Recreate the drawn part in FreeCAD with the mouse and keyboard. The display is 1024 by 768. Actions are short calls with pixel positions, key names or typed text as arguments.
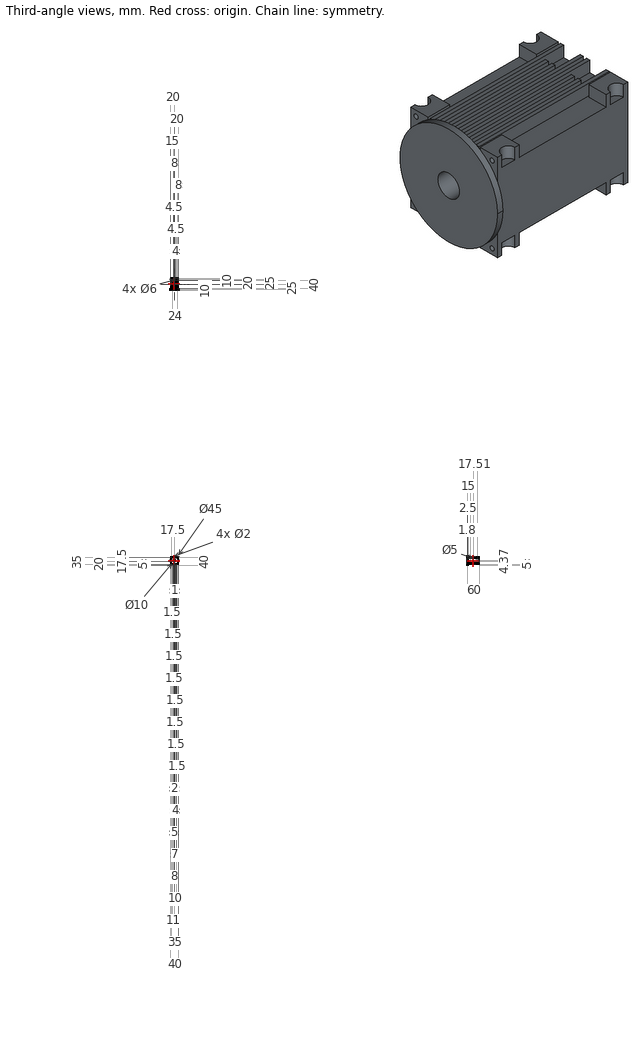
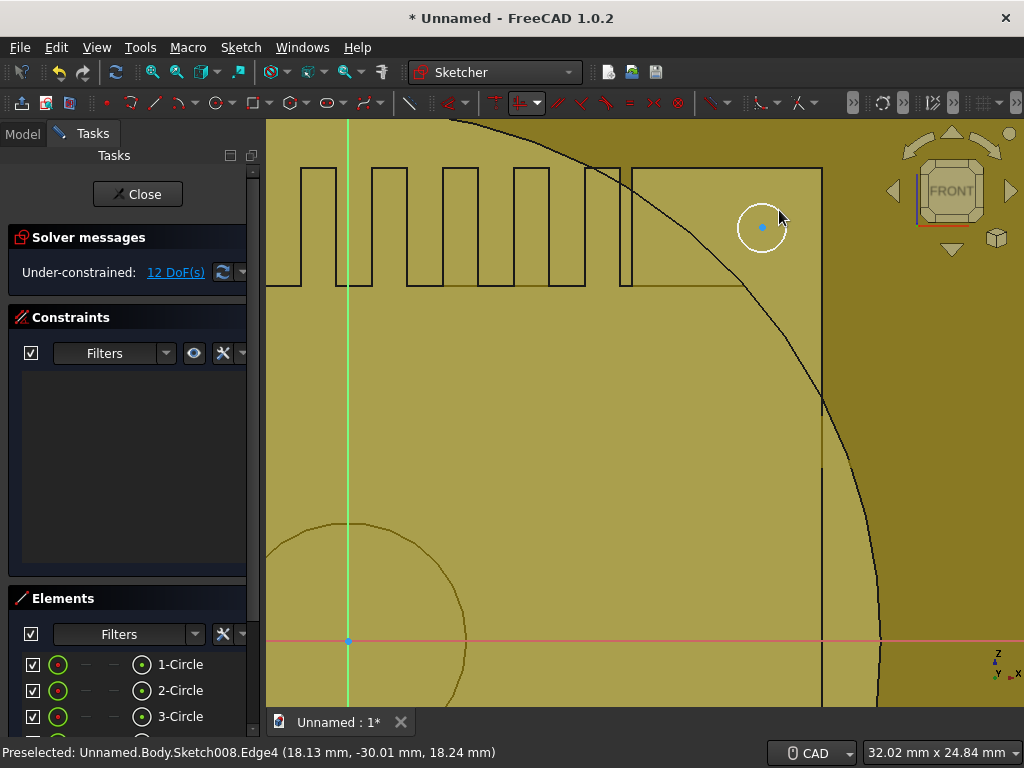
scroll(763, 227, down, 4)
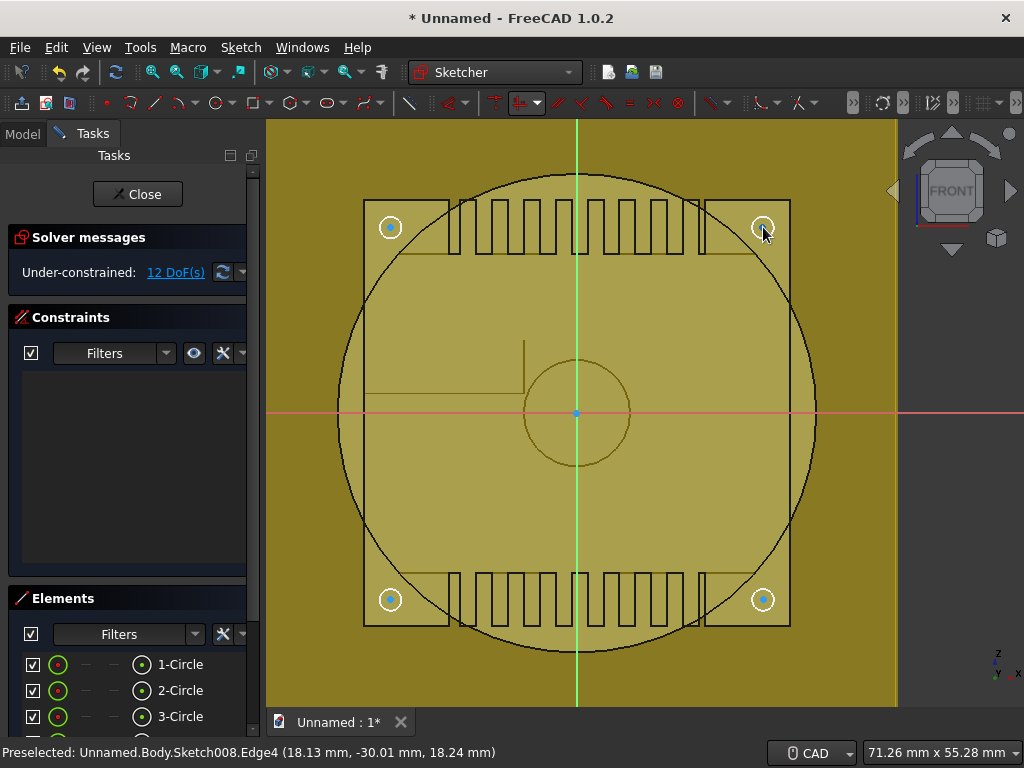
scroll(398, 220, up, 2)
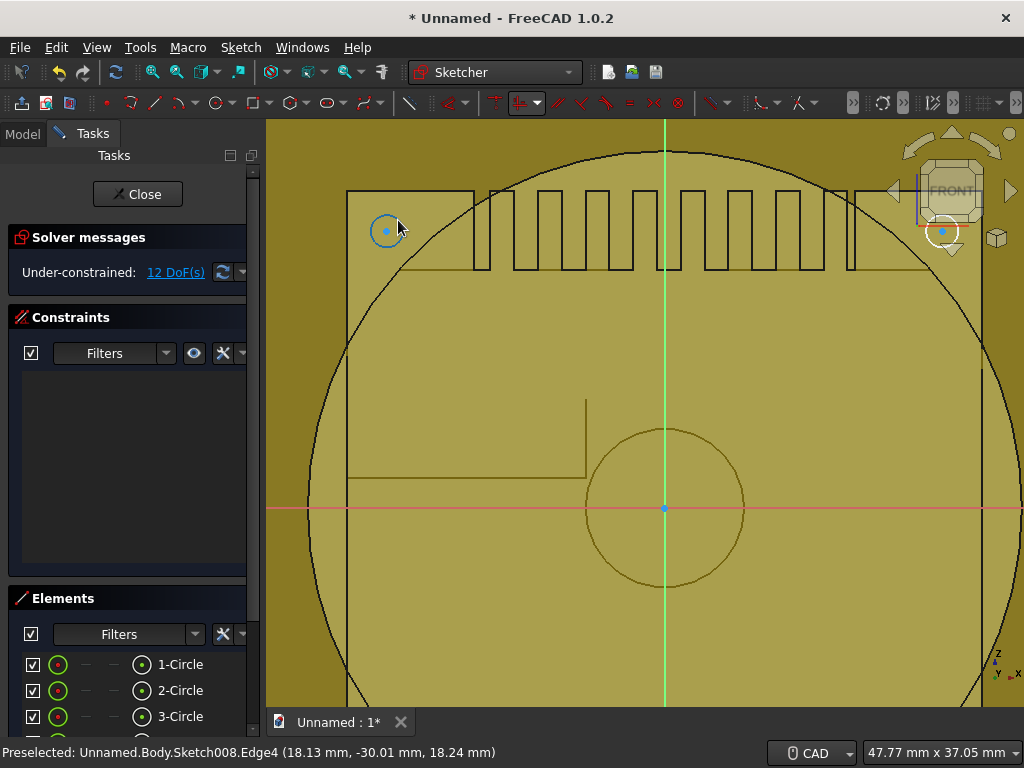
click(398, 220)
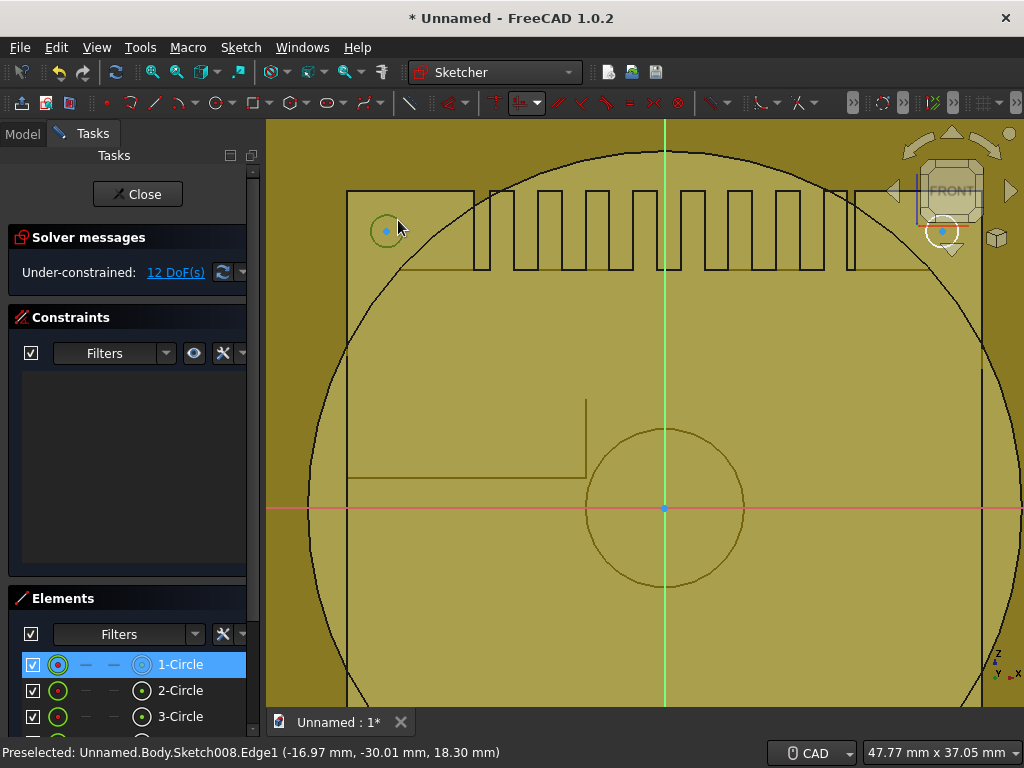
scroll(397, 220, down, 2)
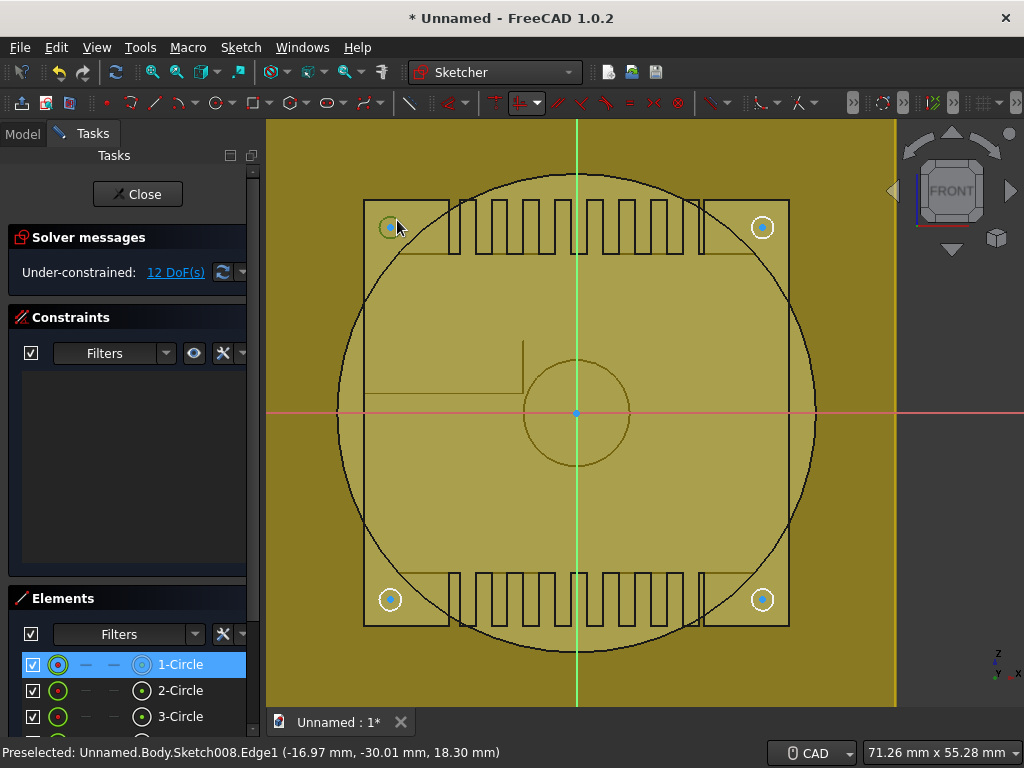
scroll(398, 592, up, 2)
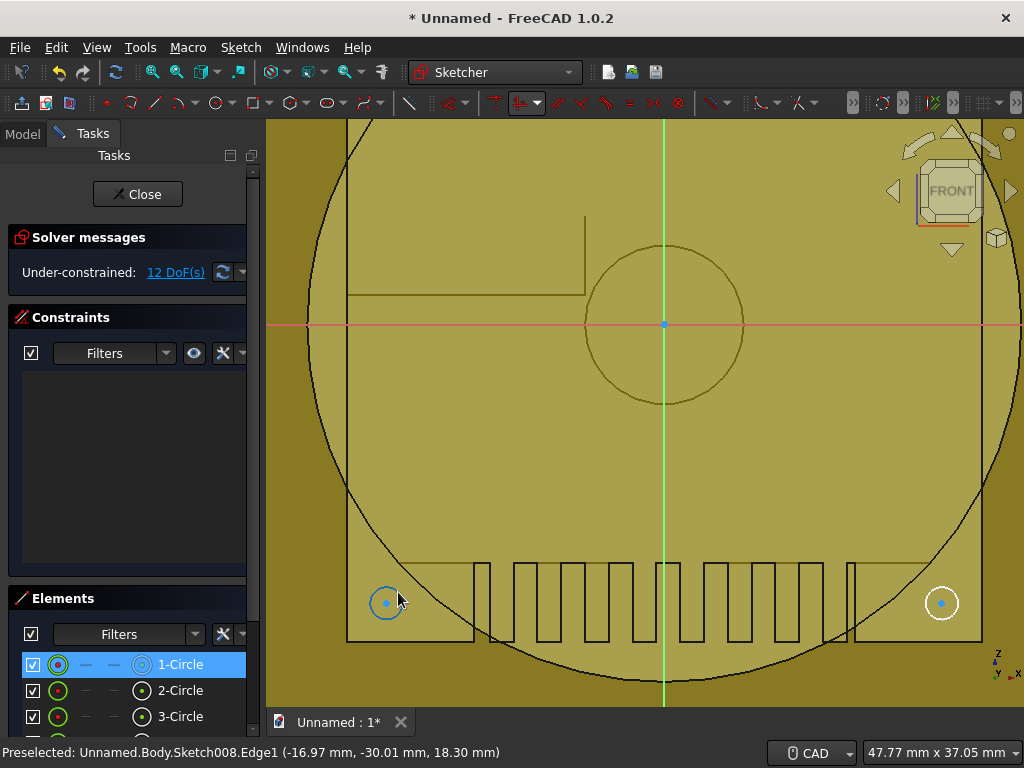
click(398, 592)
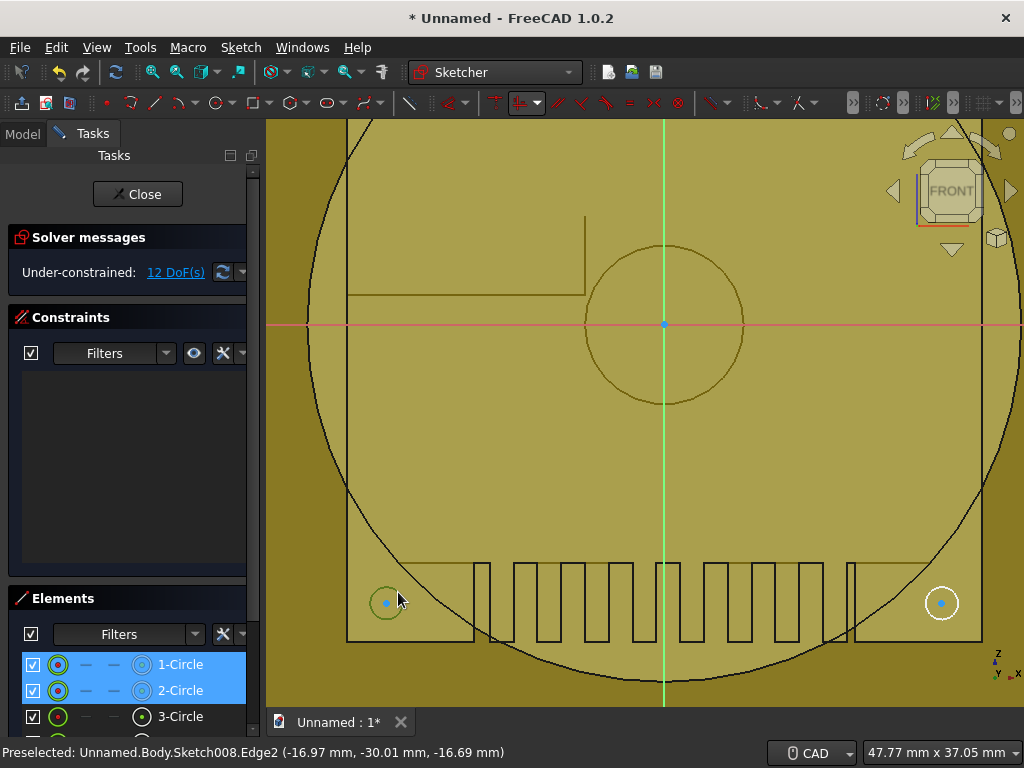
scroll(398, 592, down, 2)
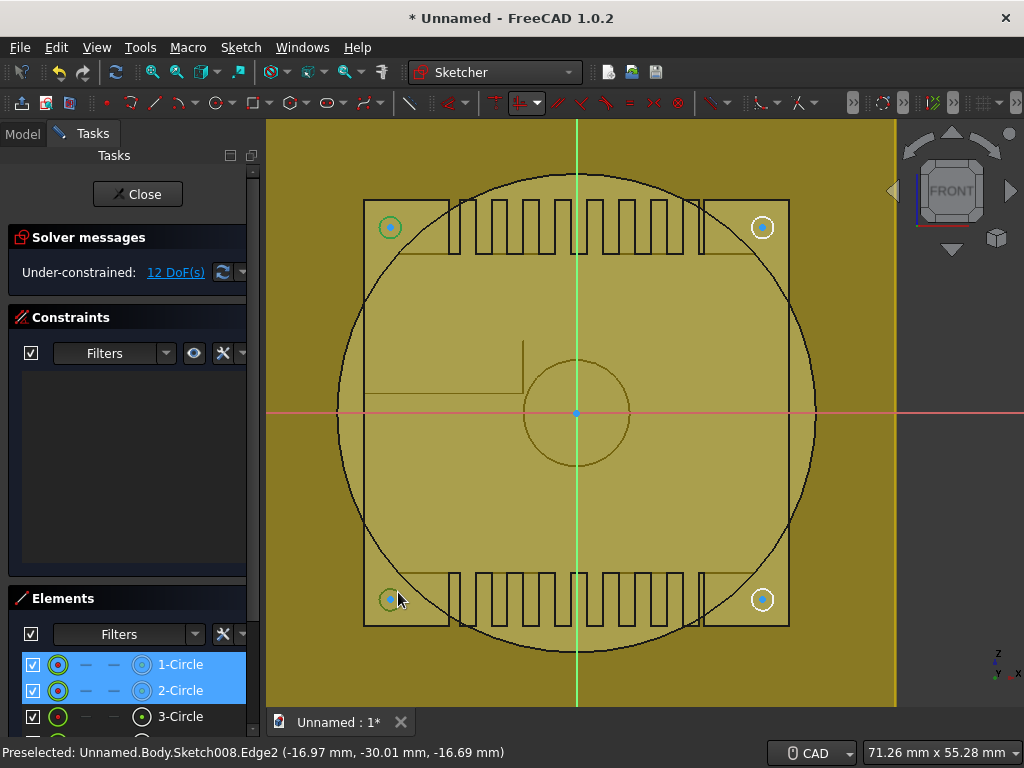
scroll(770, 592, up, 2)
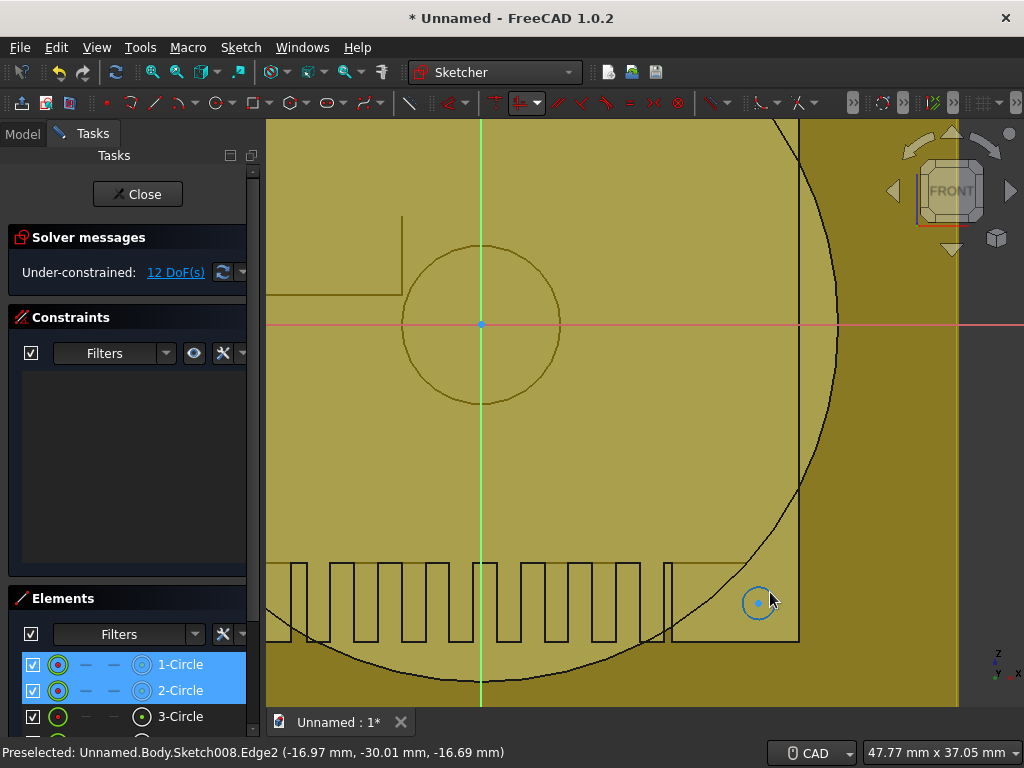
click(770, 592)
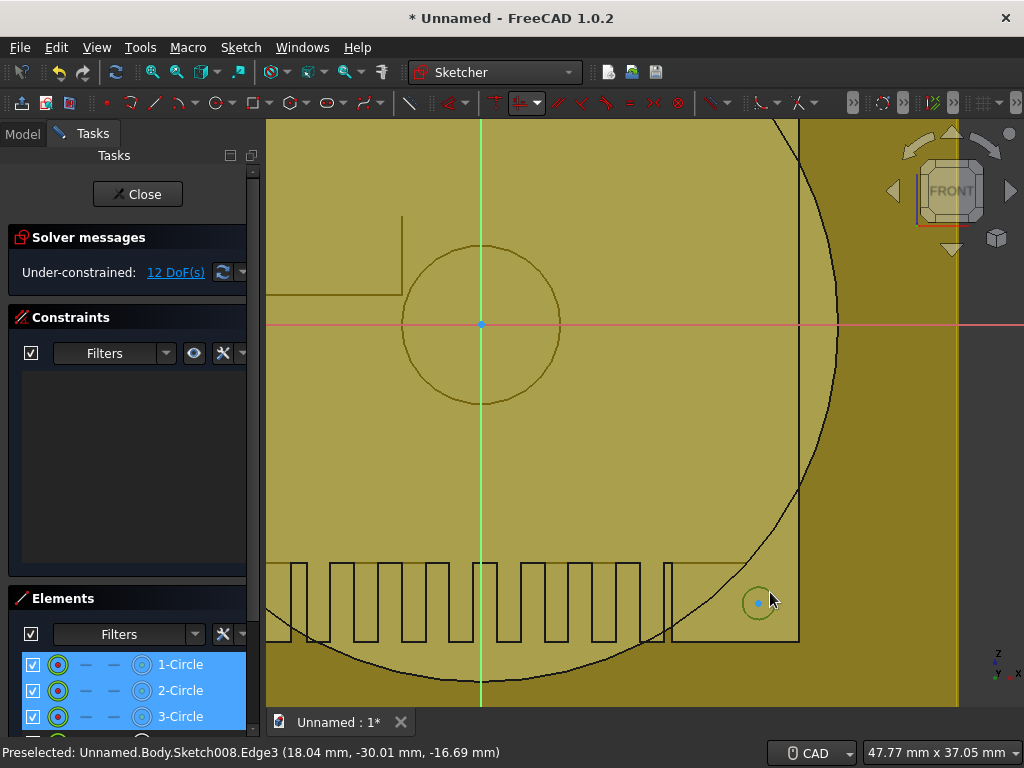
scroll(770, 592, down, 2)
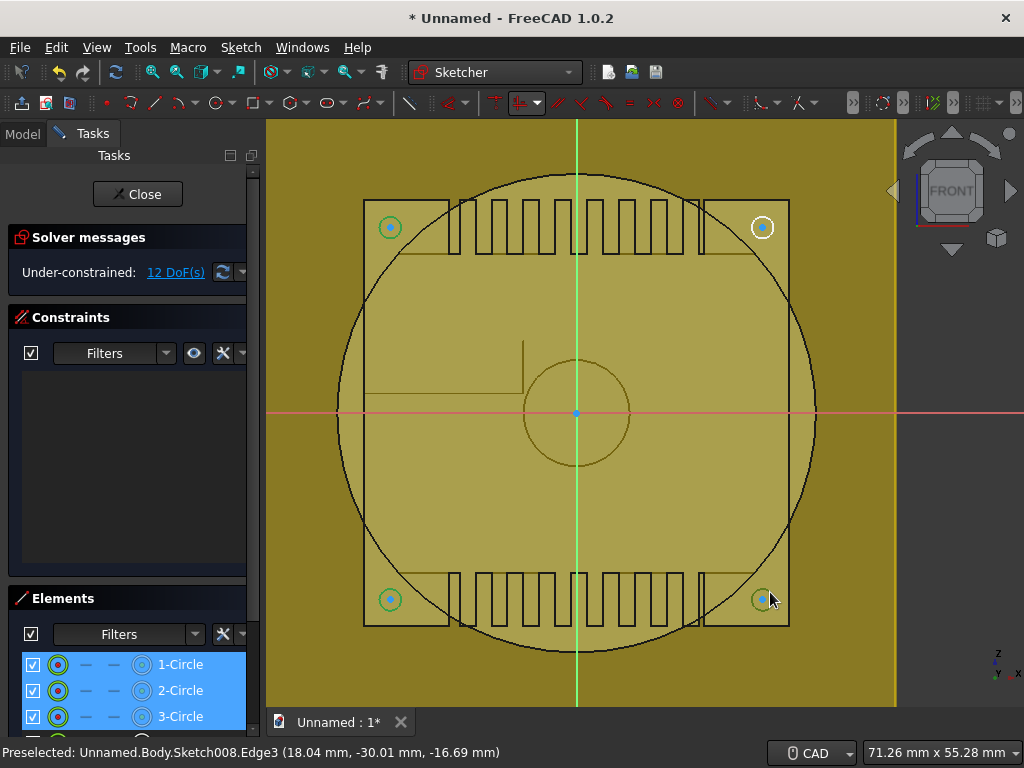
scroll(770, 220, up, 2)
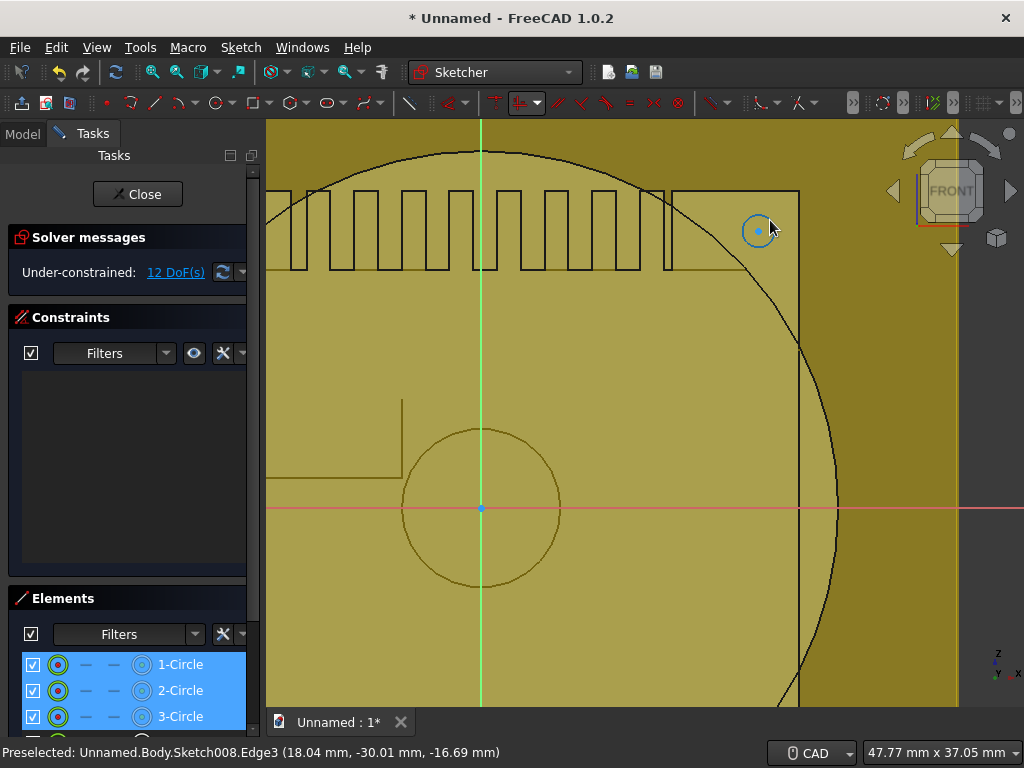
click(770, 220)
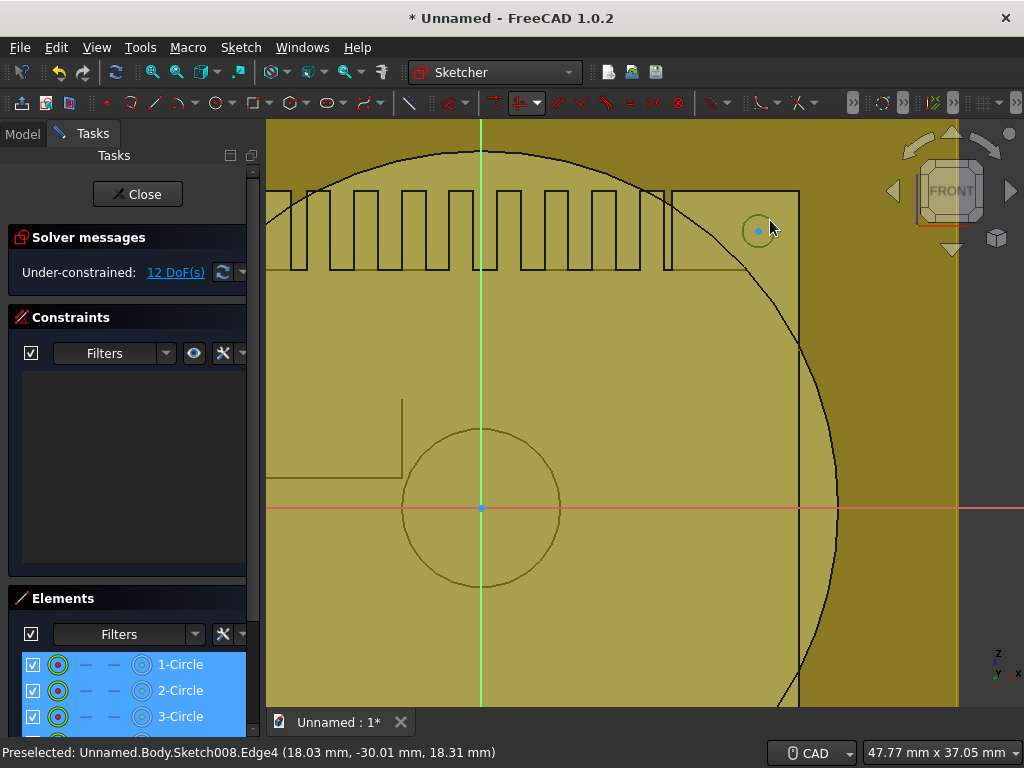
click(630, 104)